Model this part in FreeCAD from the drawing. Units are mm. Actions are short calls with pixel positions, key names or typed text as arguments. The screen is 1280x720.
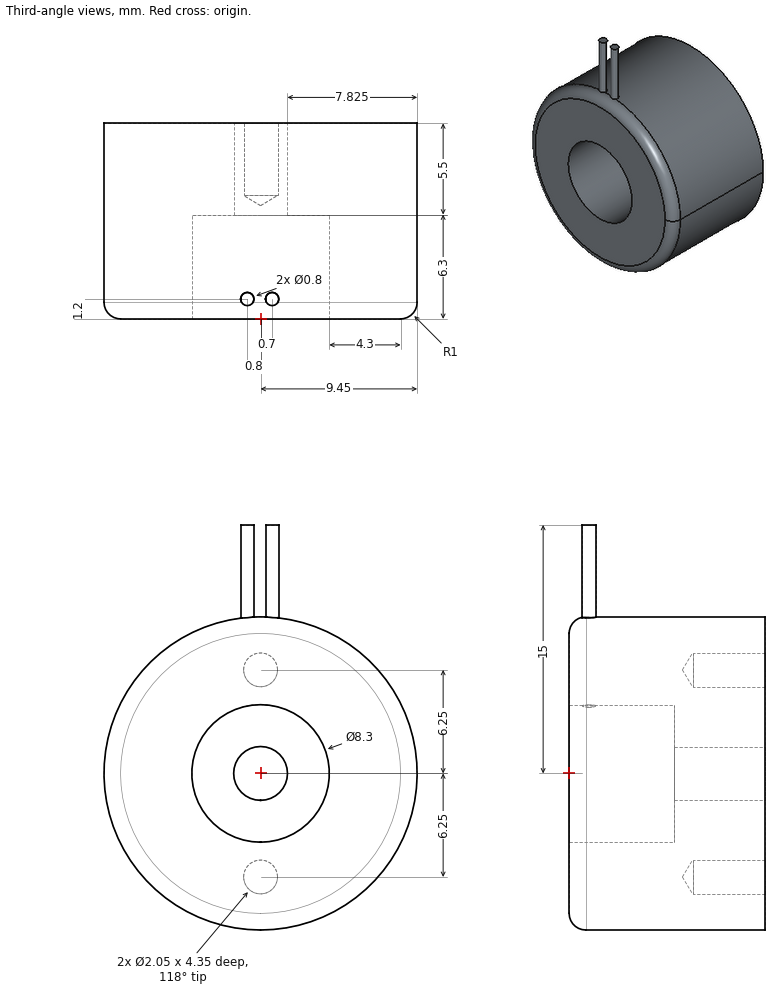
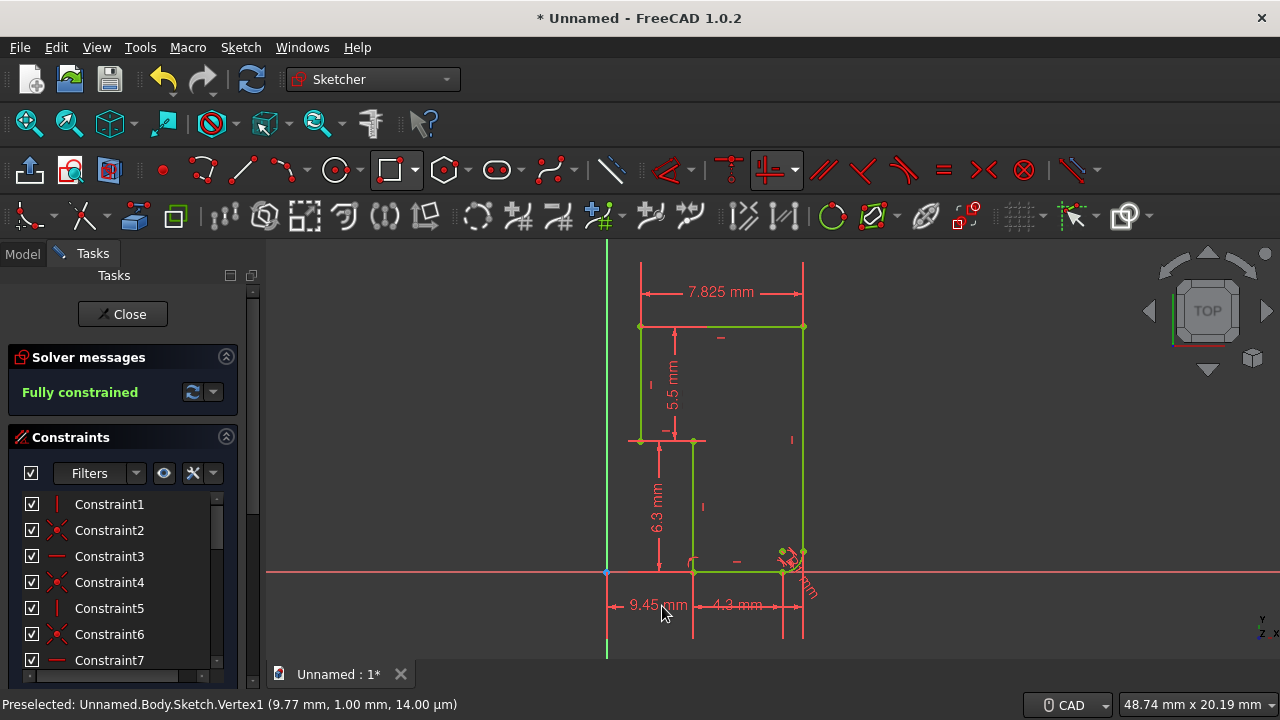
click(123, 314)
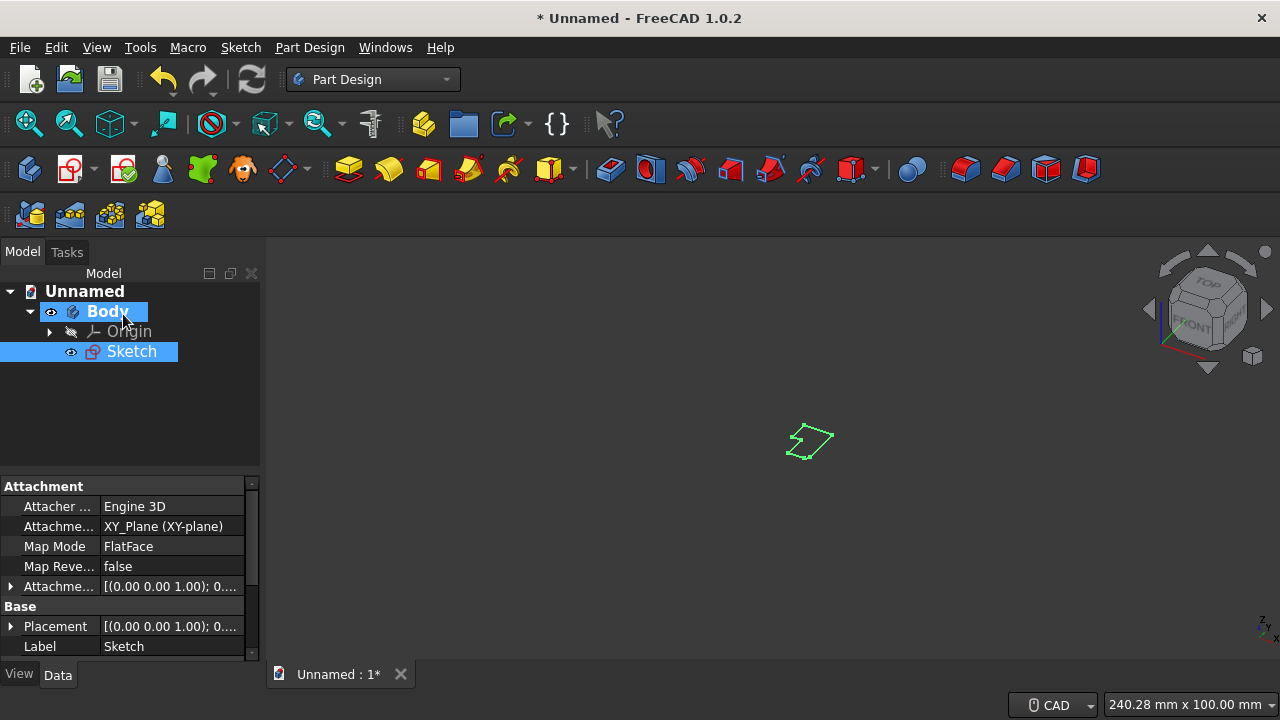
click(390, 170)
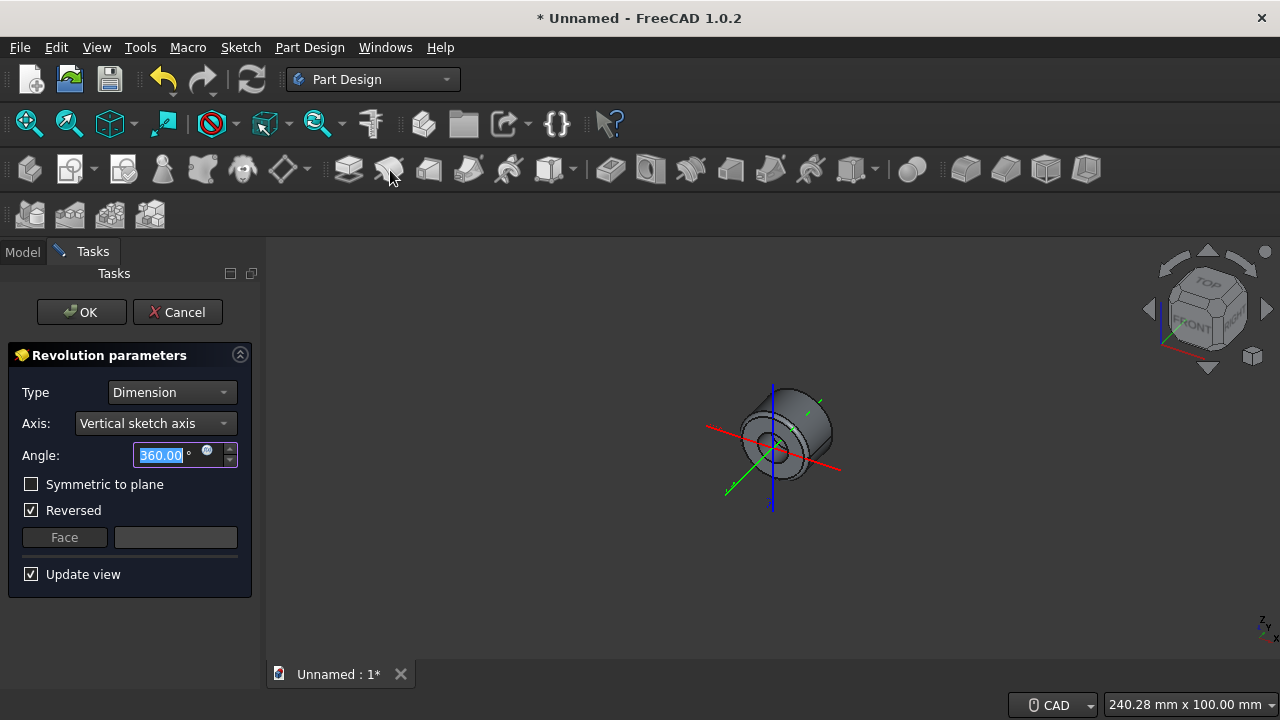
click(82, 312)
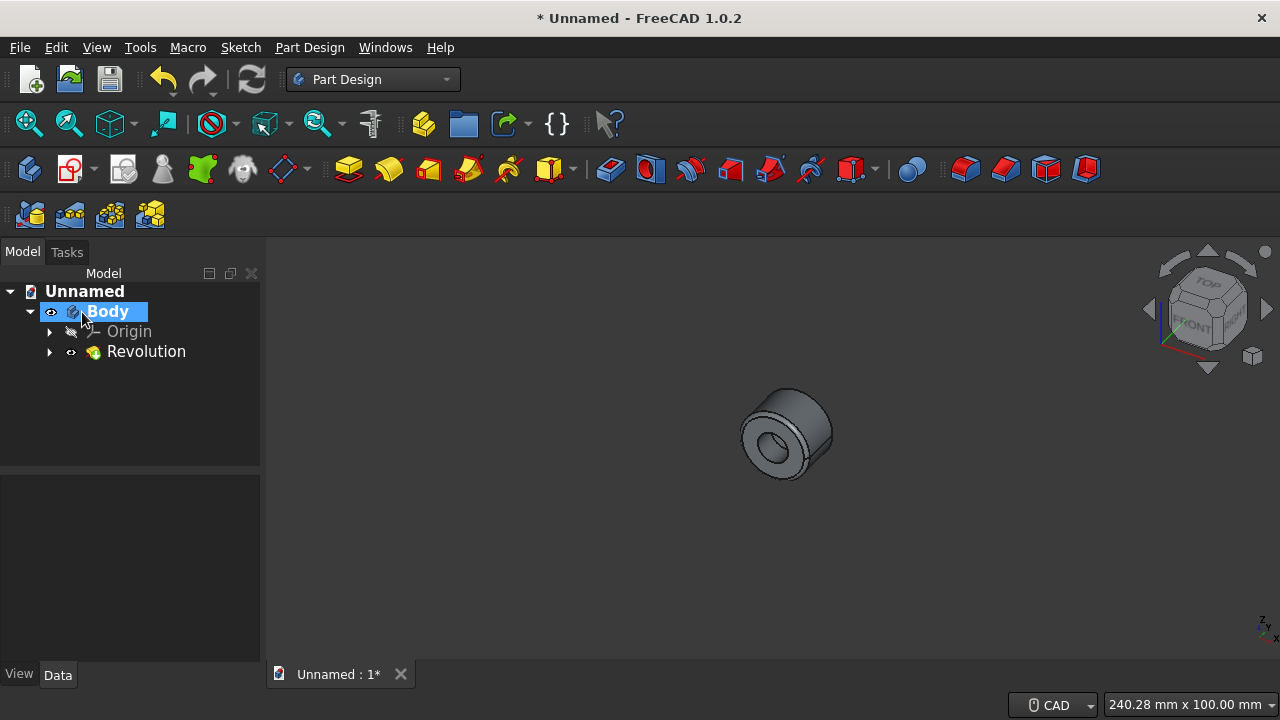
key(v)
key(f)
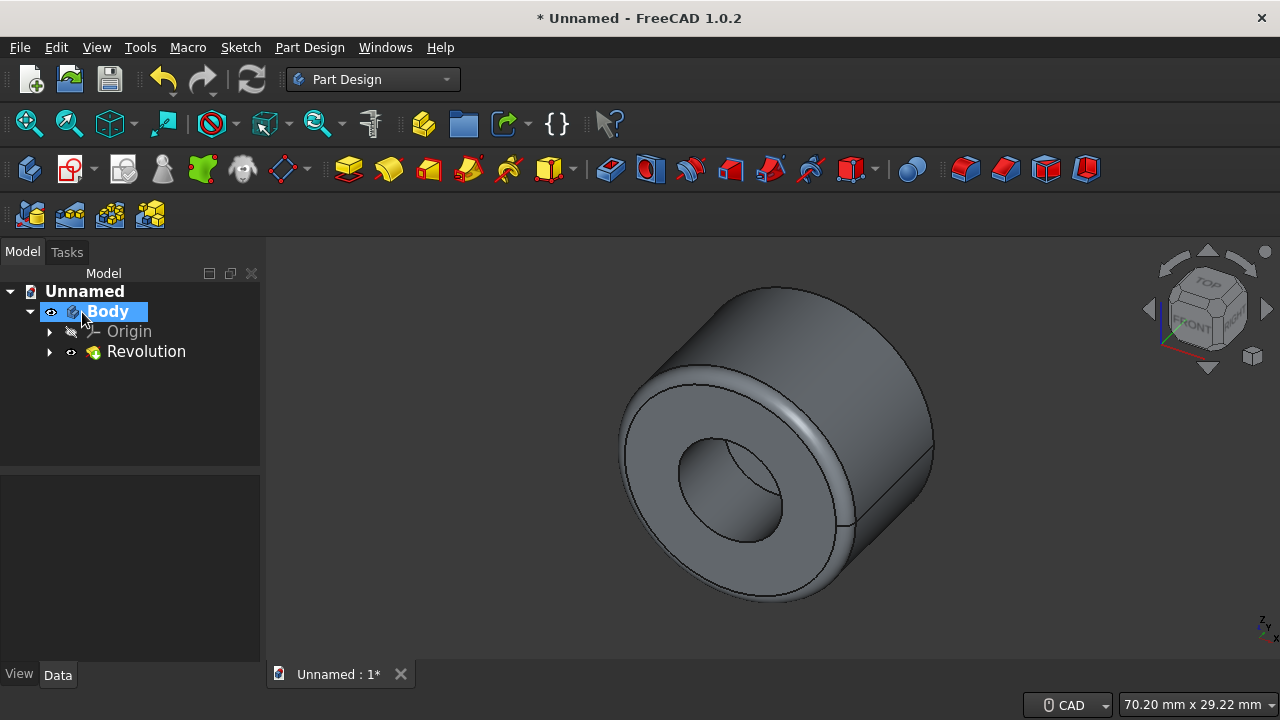
key(4)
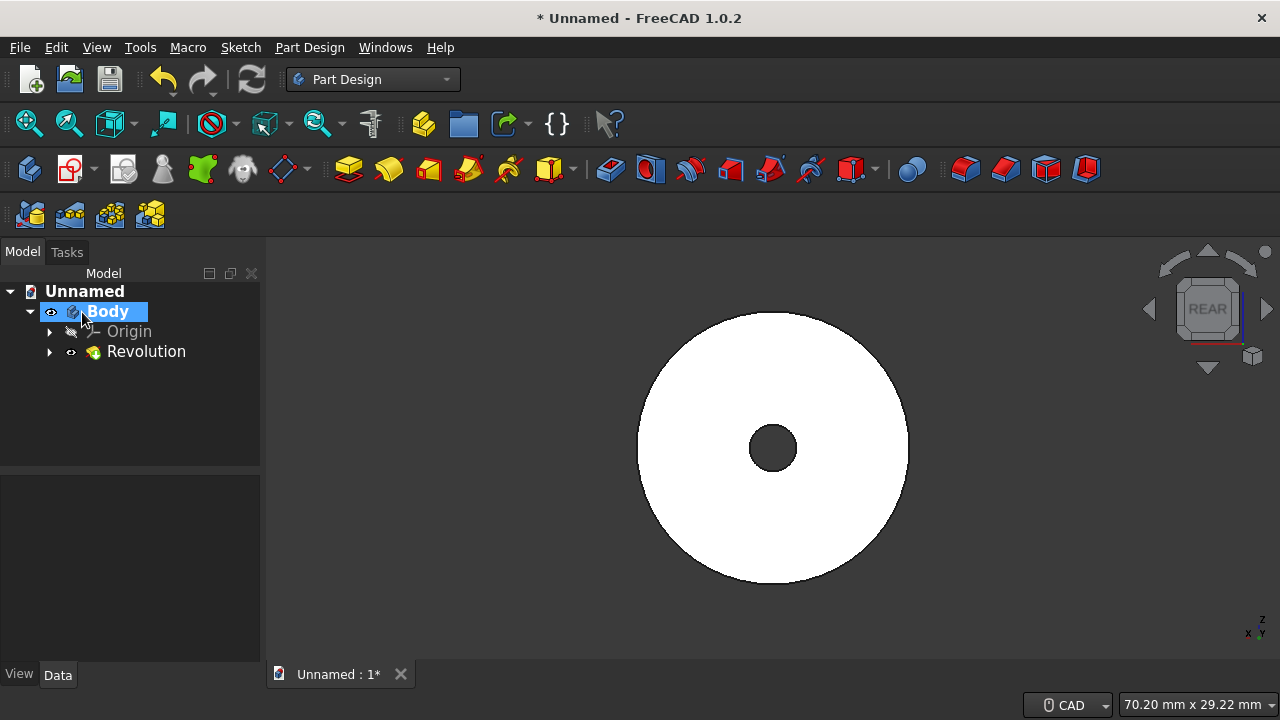
click(773, 525)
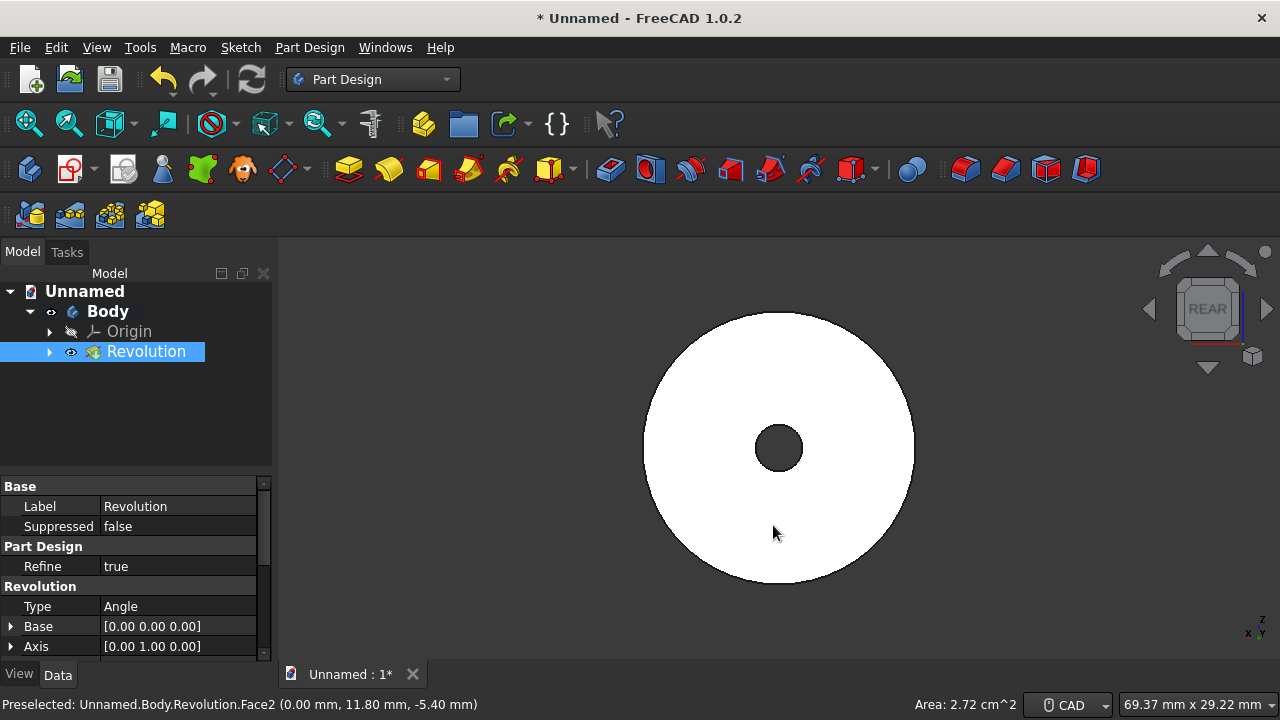
click(70, 170)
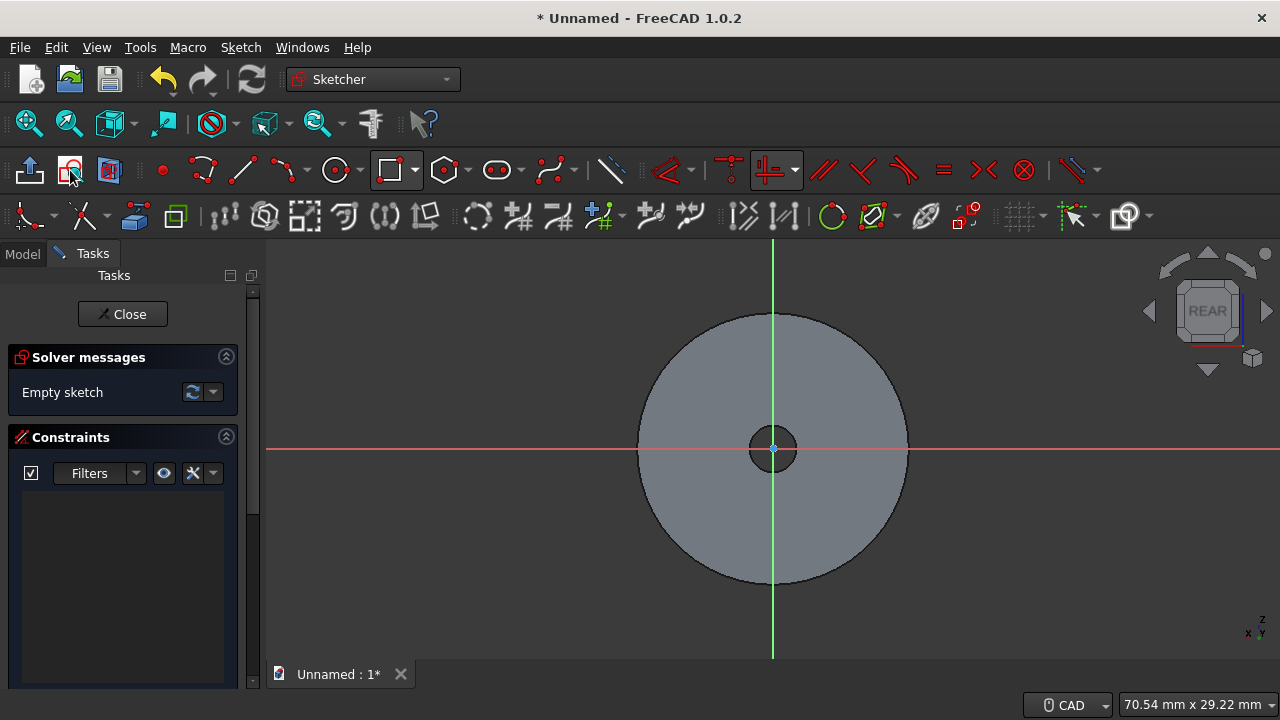
key(g)
key(c)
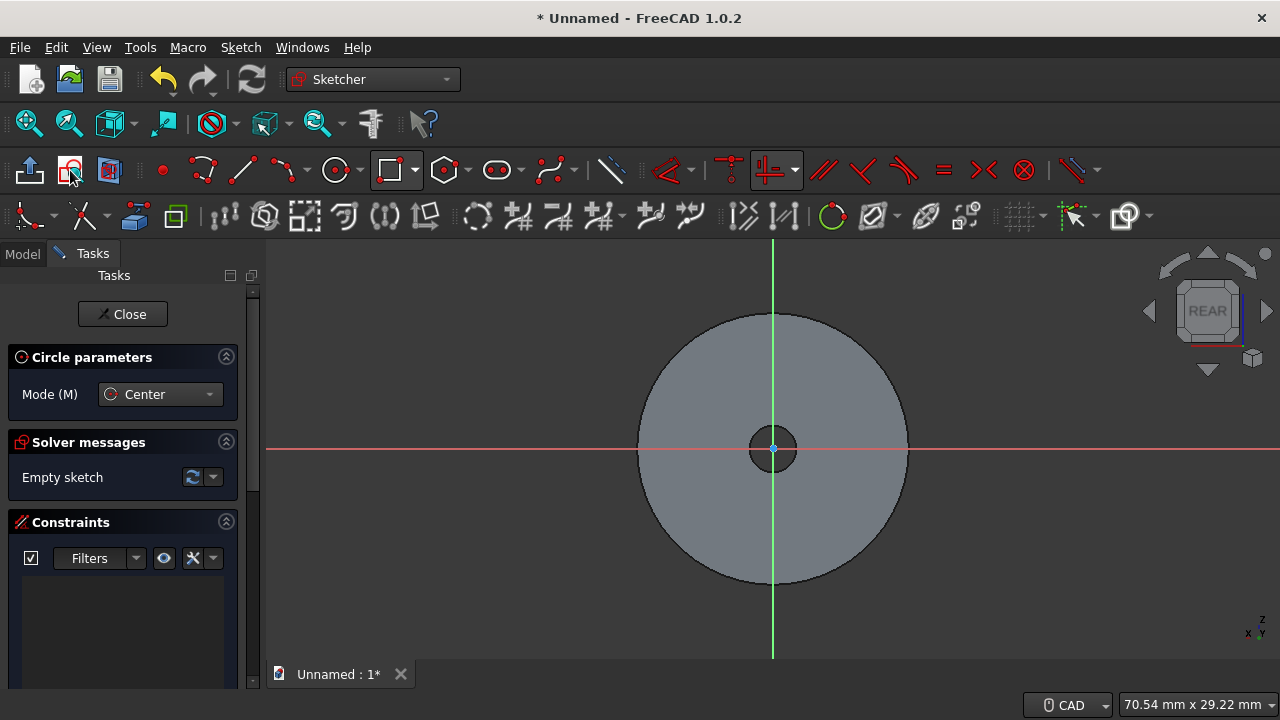
scroll(773, 539, up, 3)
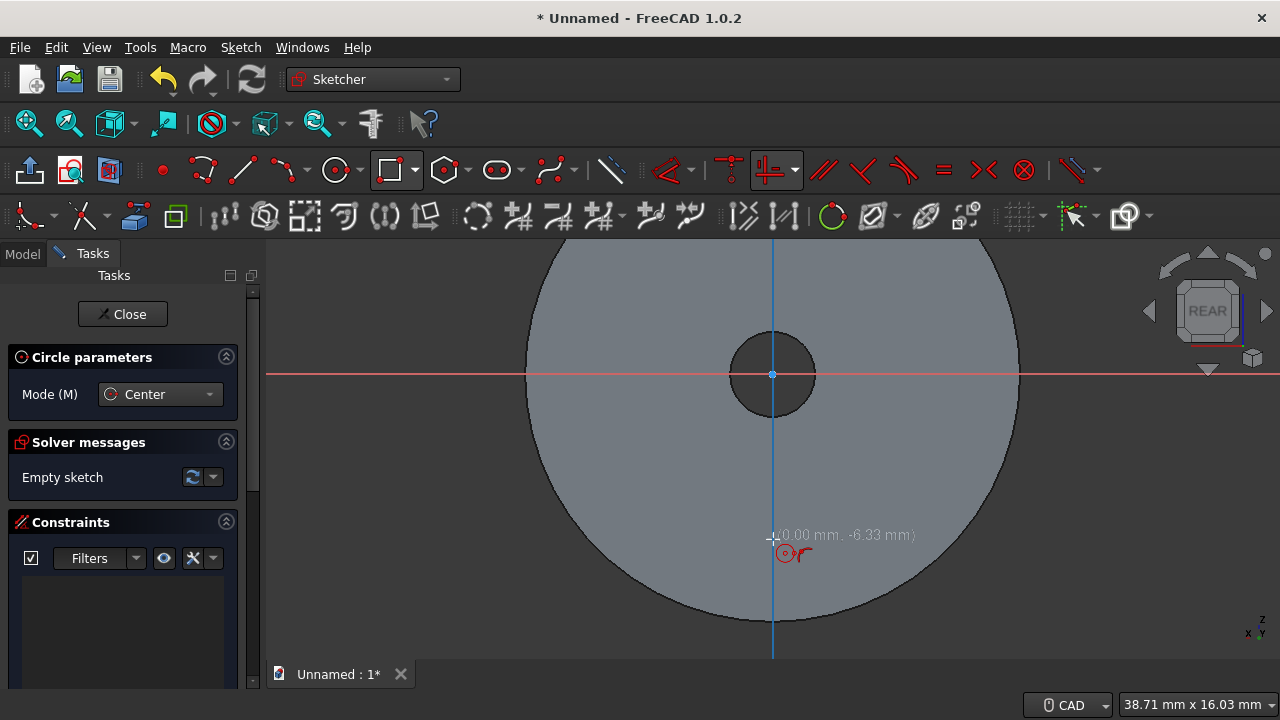
click(773, 538)
move(792, 519)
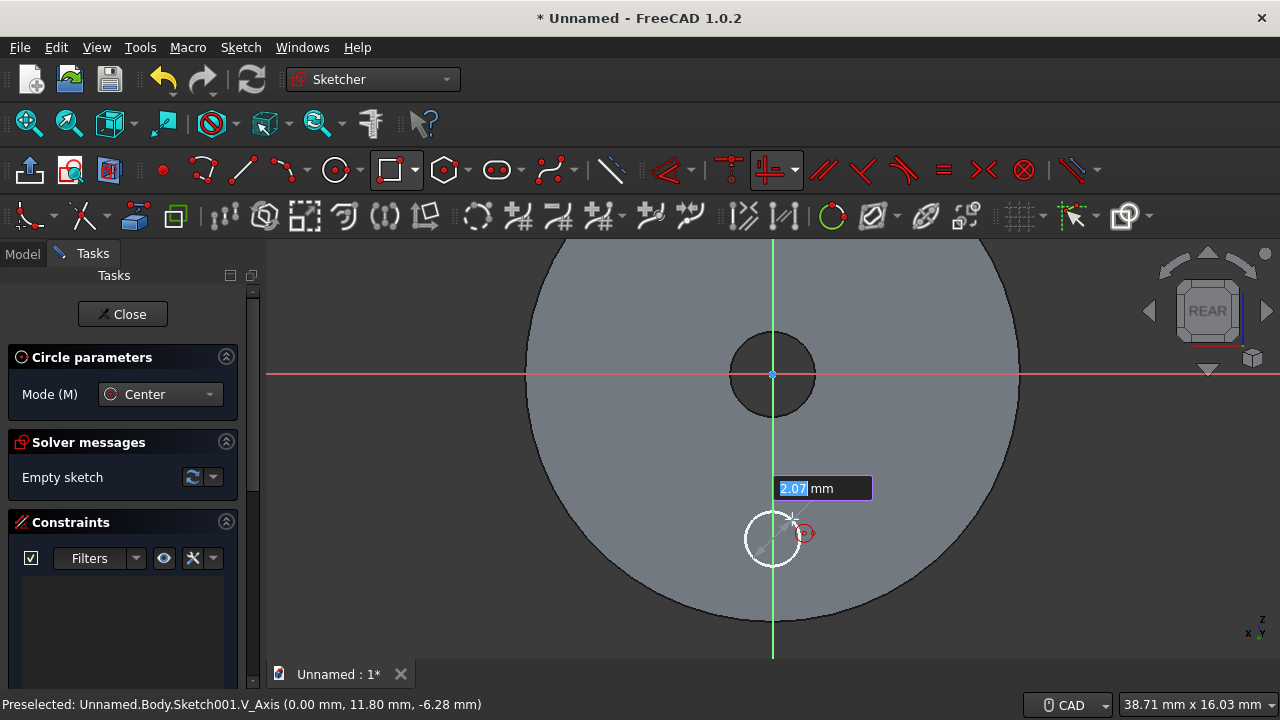
text(2.05)
key(Return)